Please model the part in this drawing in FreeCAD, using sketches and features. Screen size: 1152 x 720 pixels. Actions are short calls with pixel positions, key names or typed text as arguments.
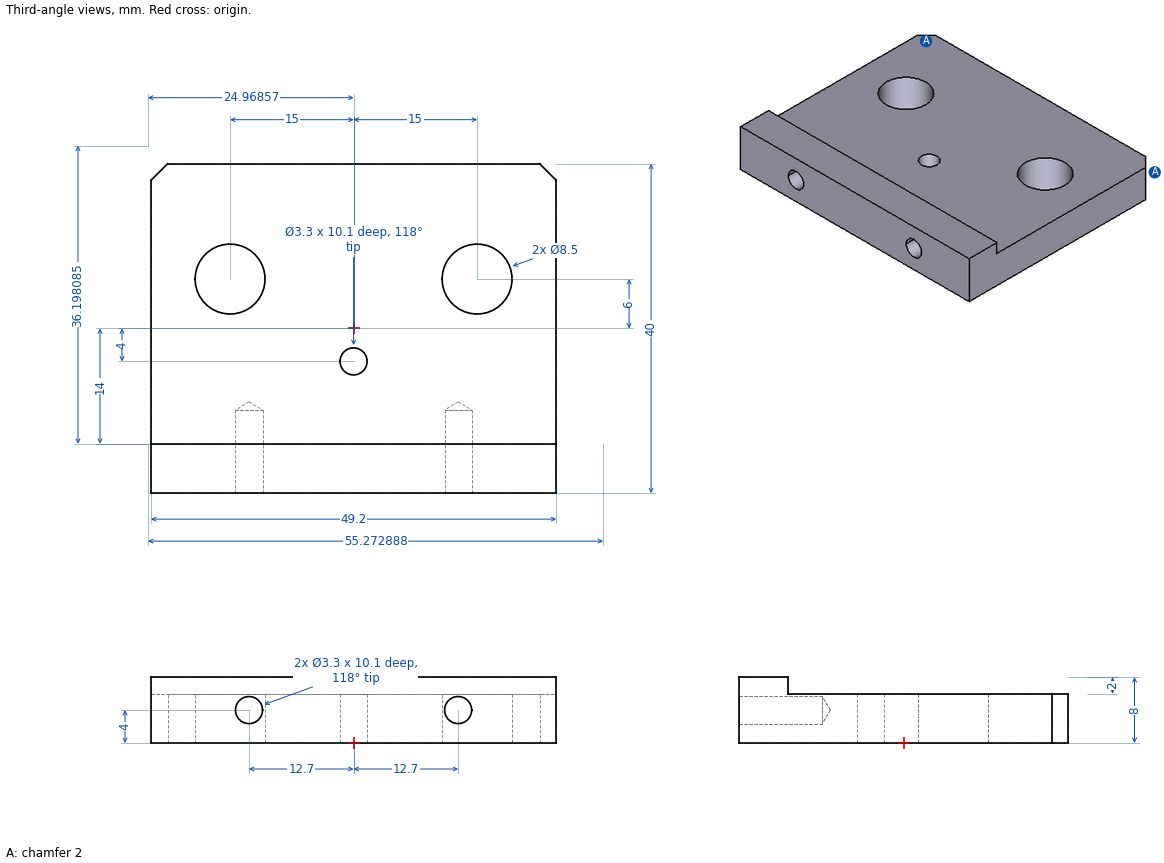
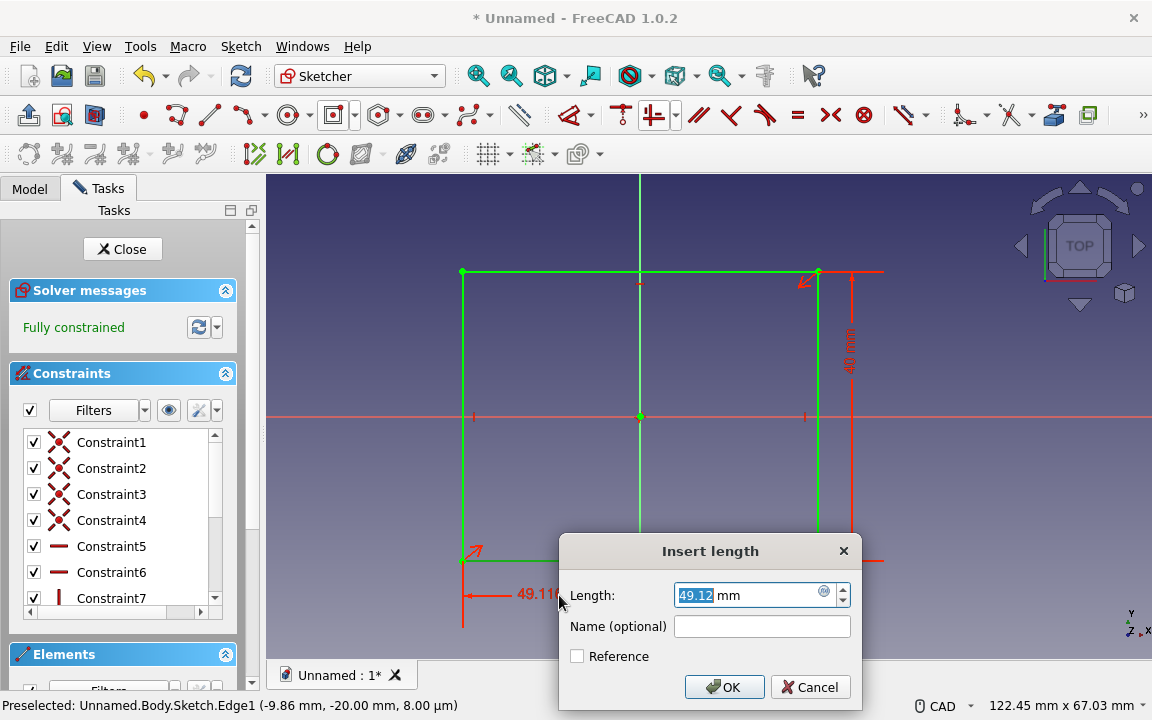
text(49.2)
key(Return)
key(Escape)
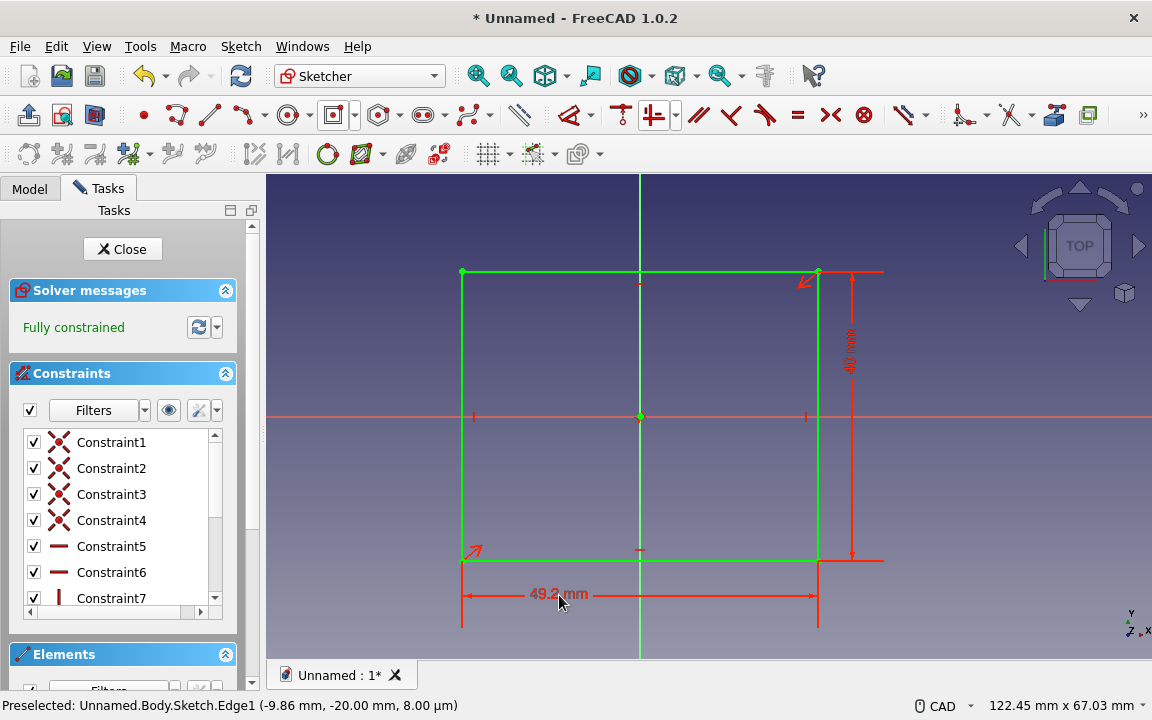
click(123, 249)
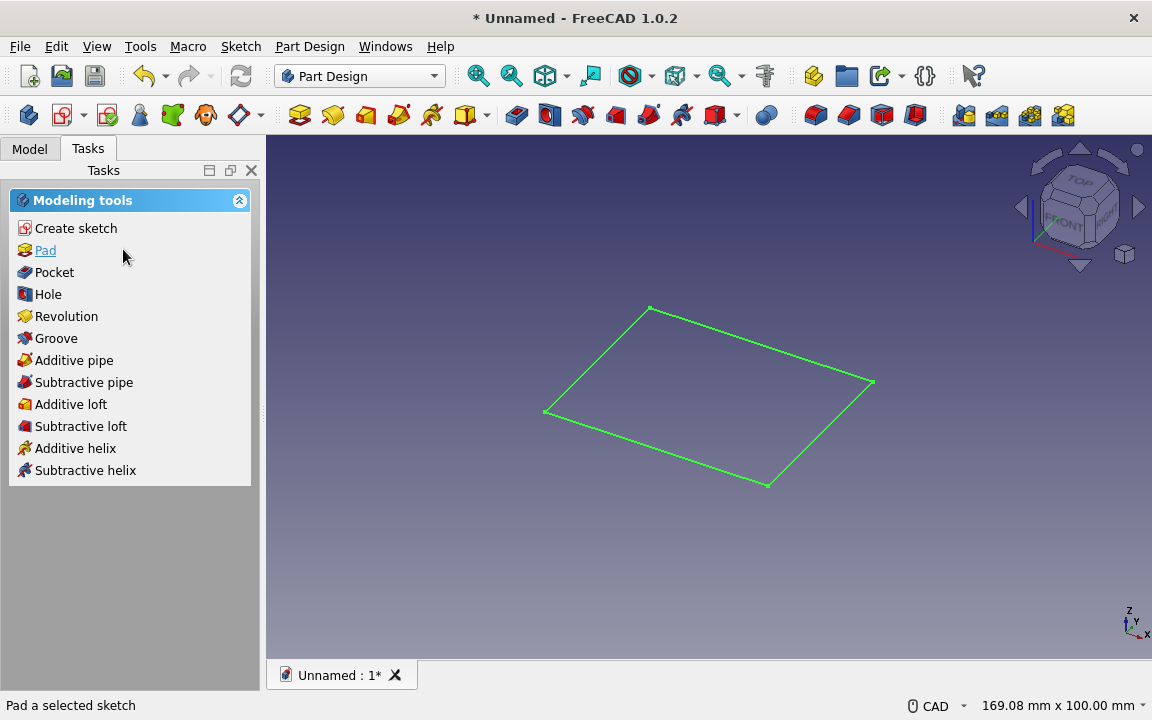
click(300, 116)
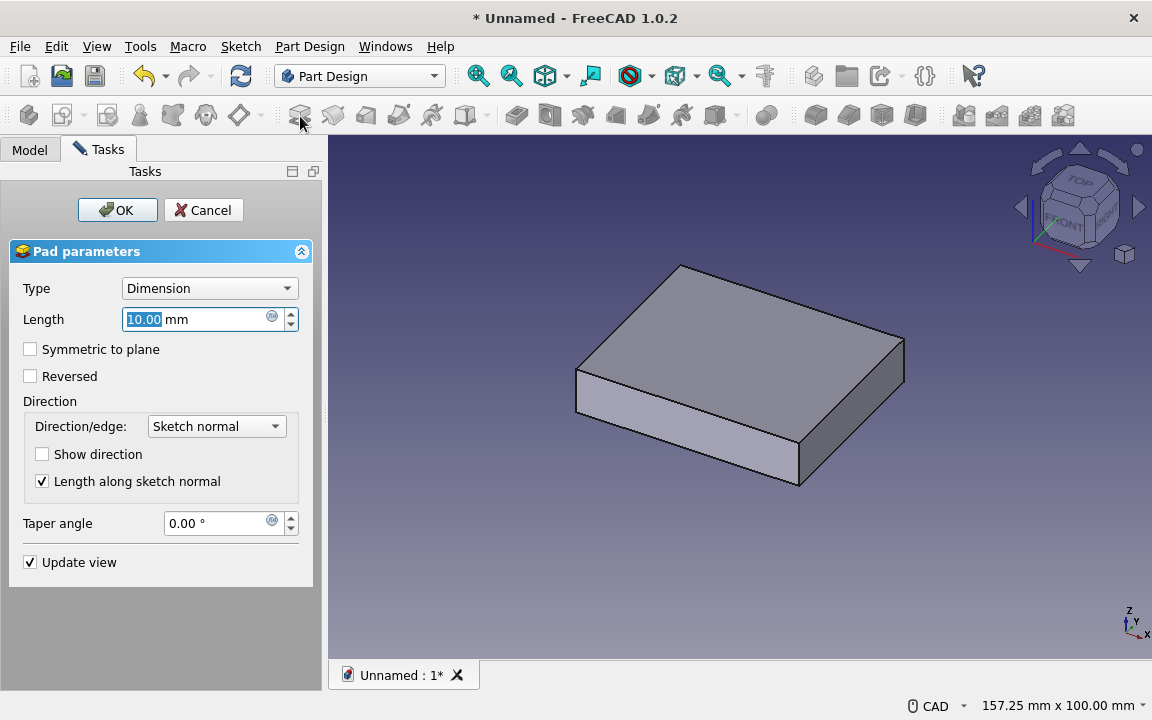
text(8)
key(Tab)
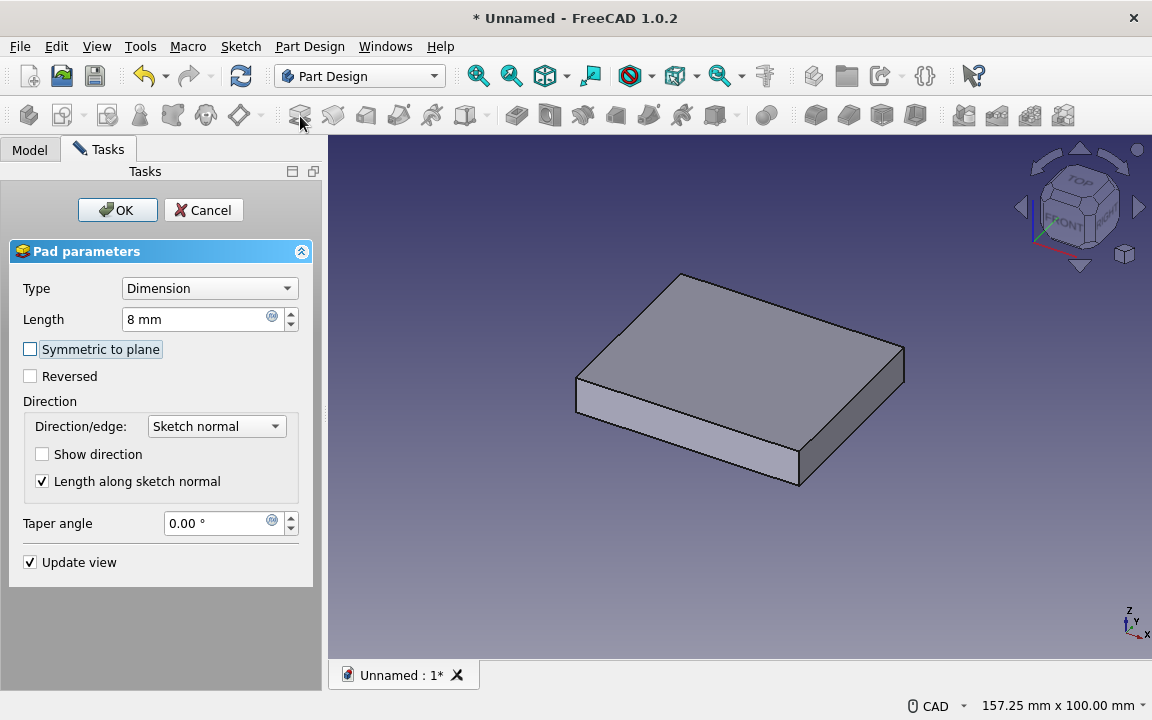
click(118, 210)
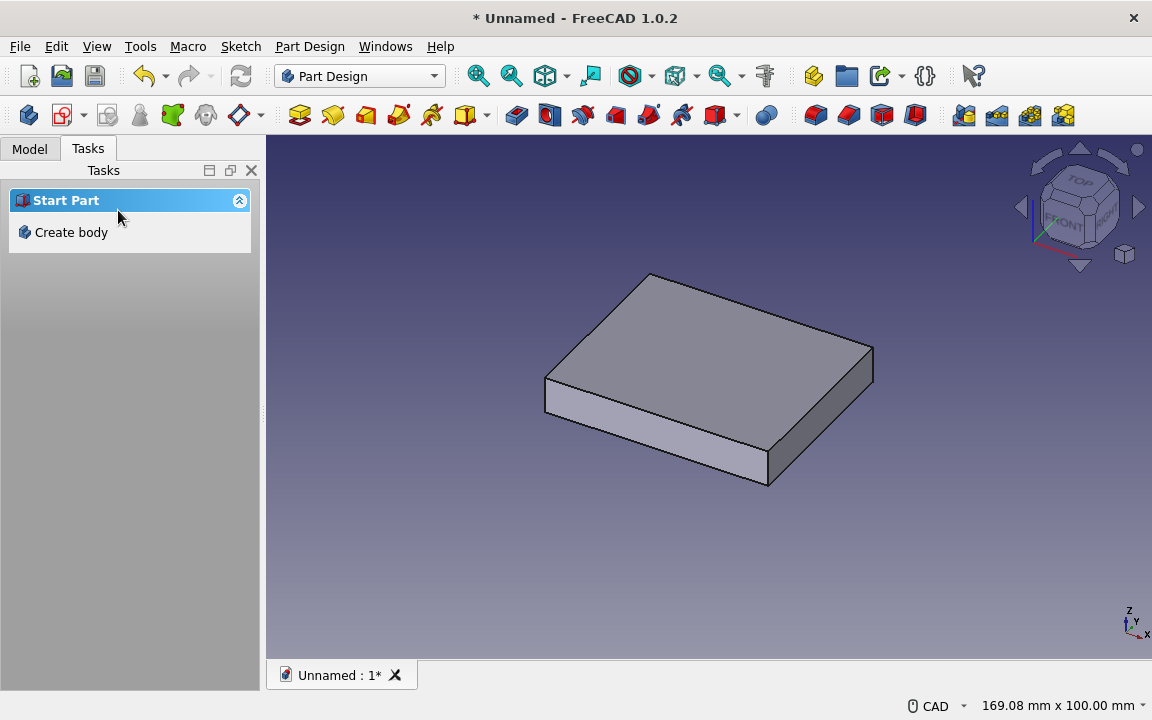
key(v)
key(f)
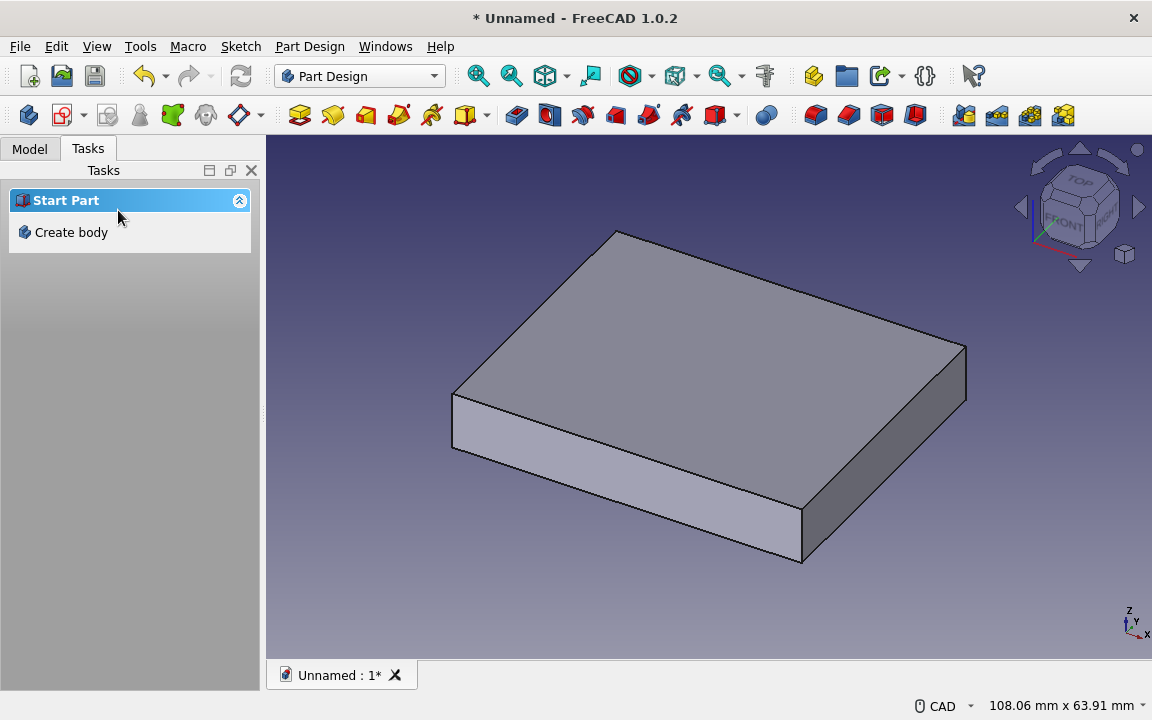
click(727, 511)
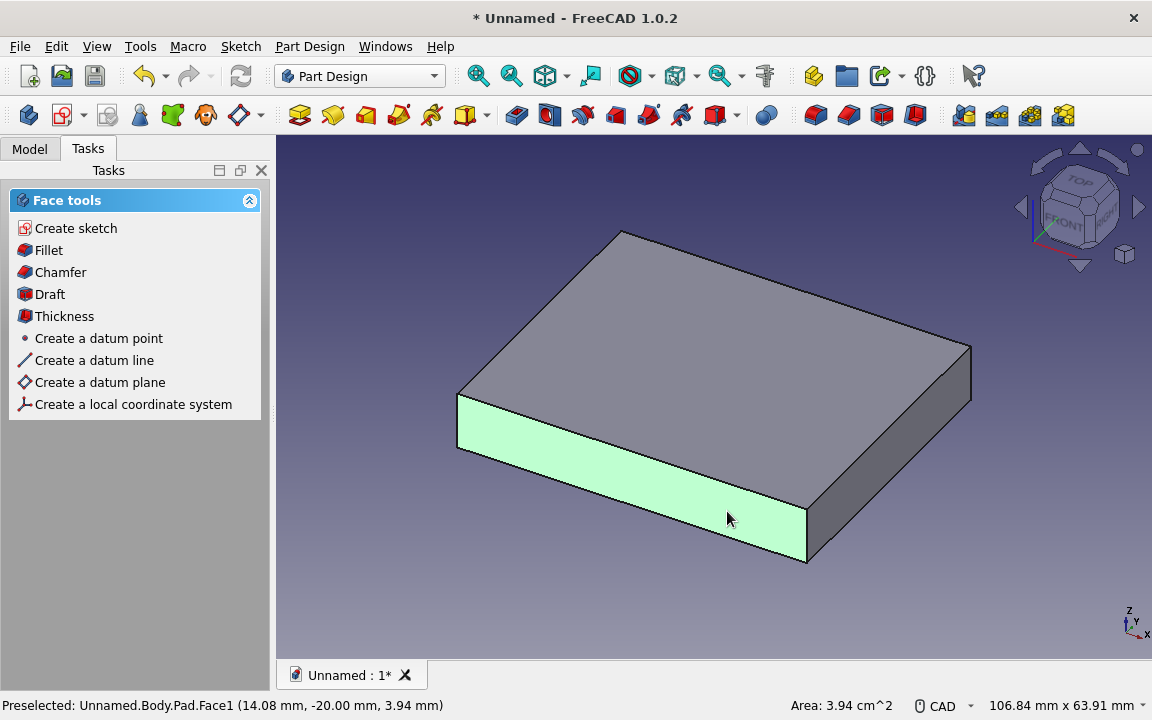
click(62, 116)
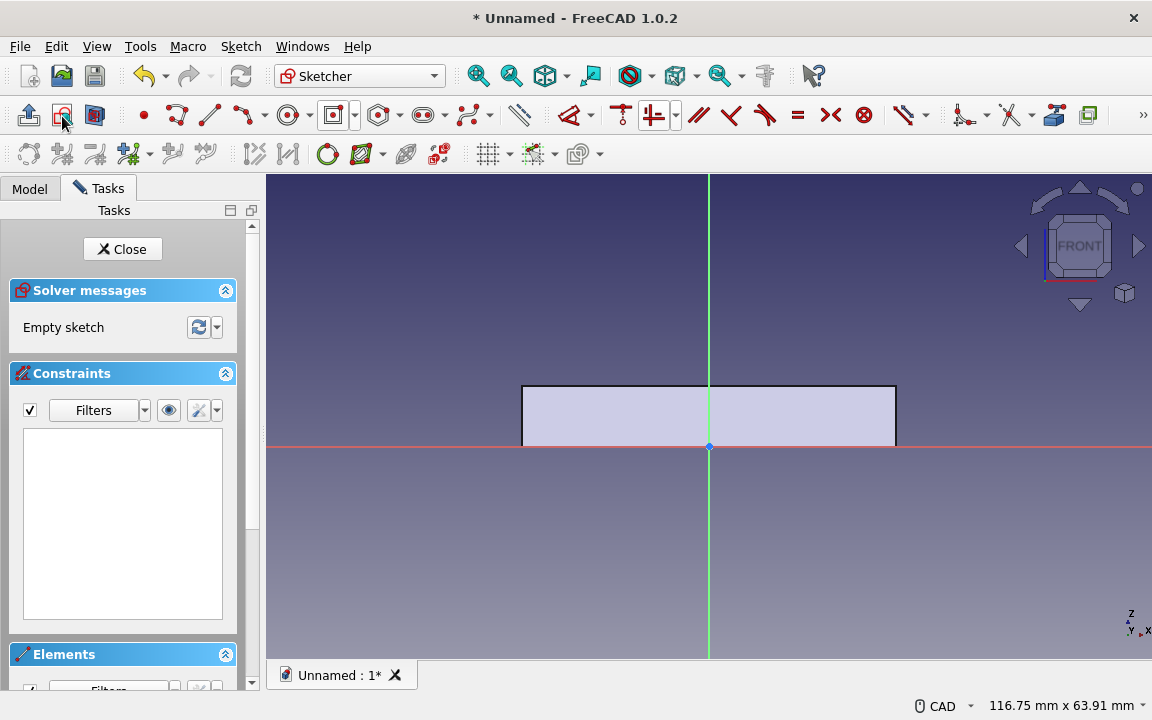
scroll(765, 433, up, 4)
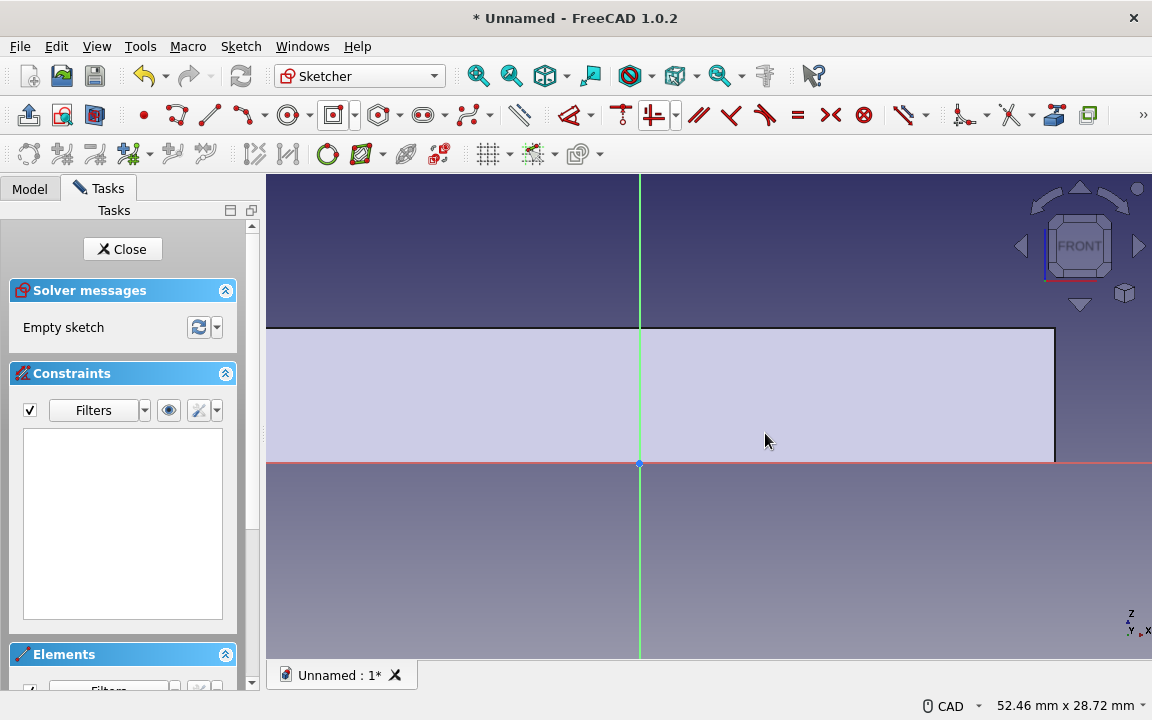
key(g)
key(c)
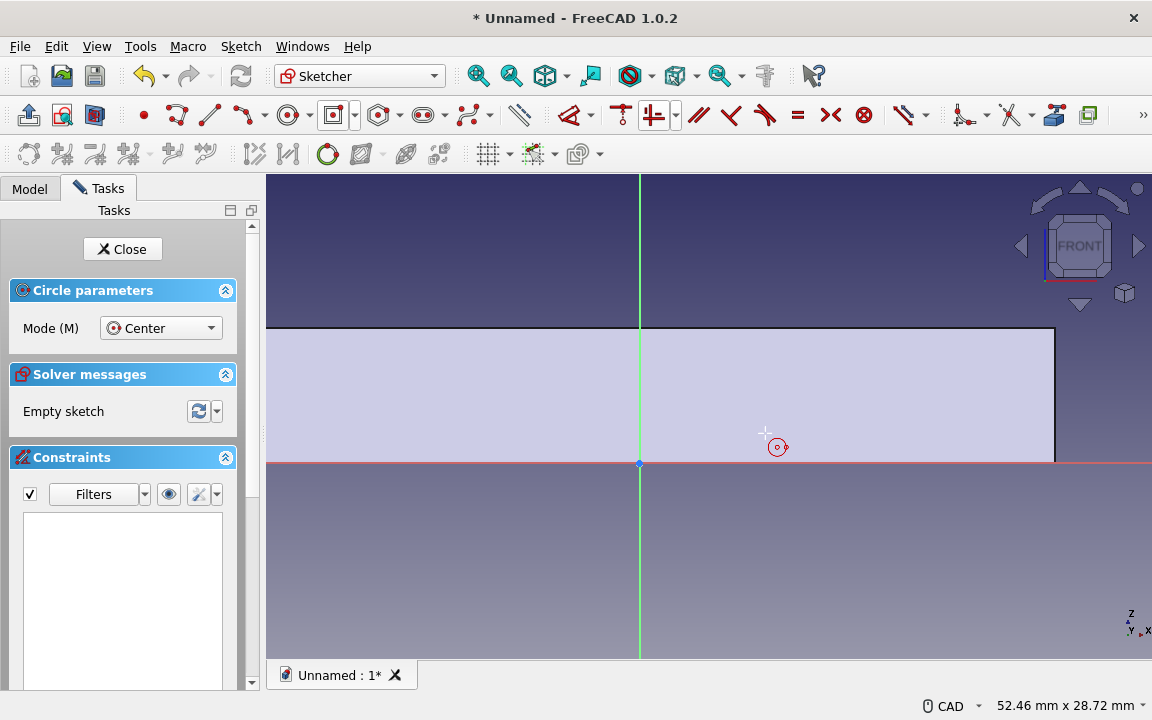
click(425, 396)
click(445, 376)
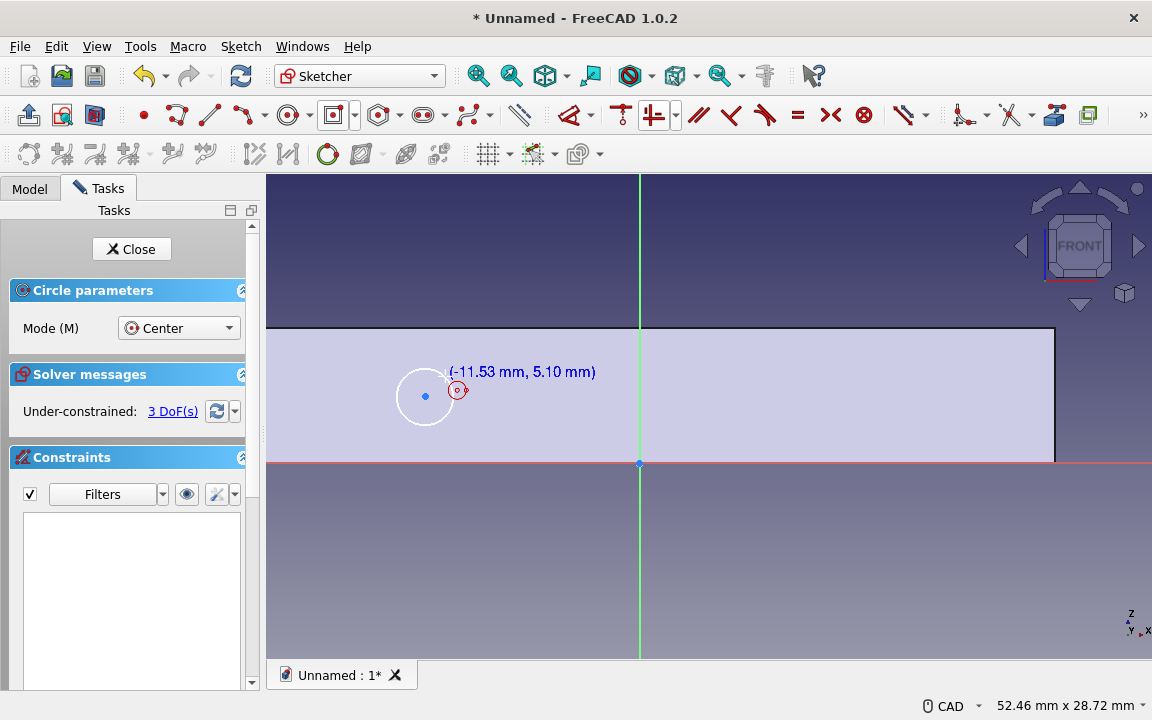
click(854, 396)
click(874, 376)
key(Escape)